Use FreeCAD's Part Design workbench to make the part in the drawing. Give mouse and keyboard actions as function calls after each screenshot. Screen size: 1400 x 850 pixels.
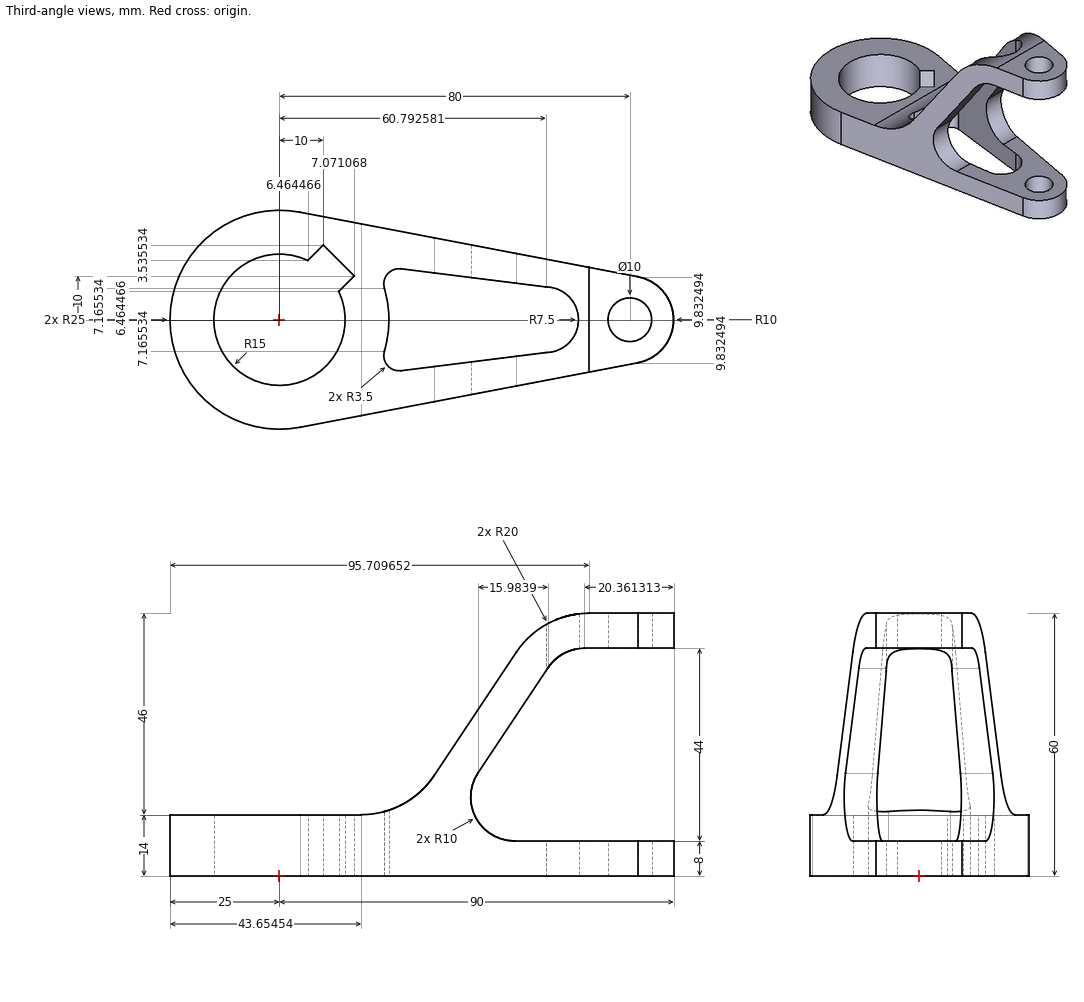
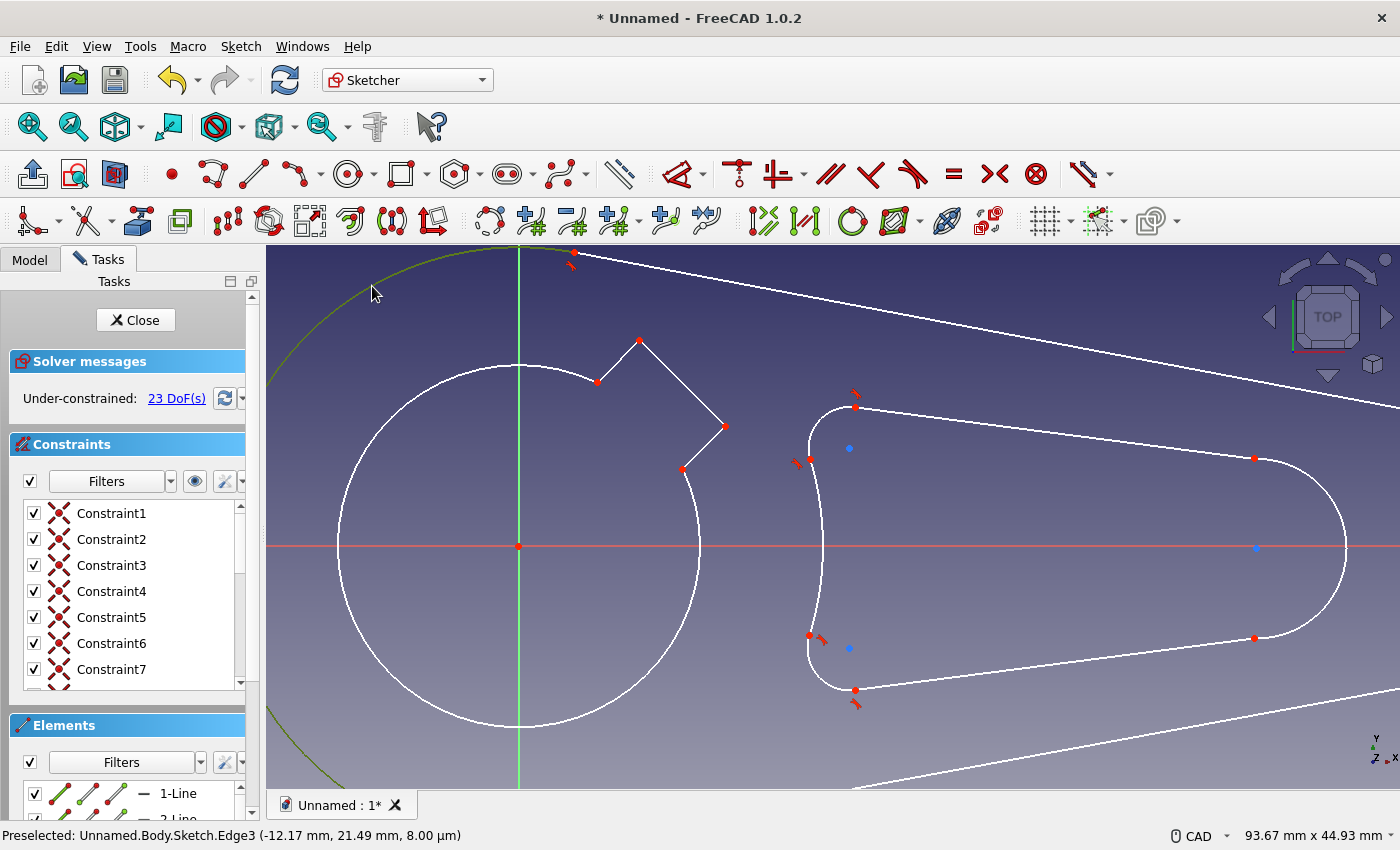
click(821, 583)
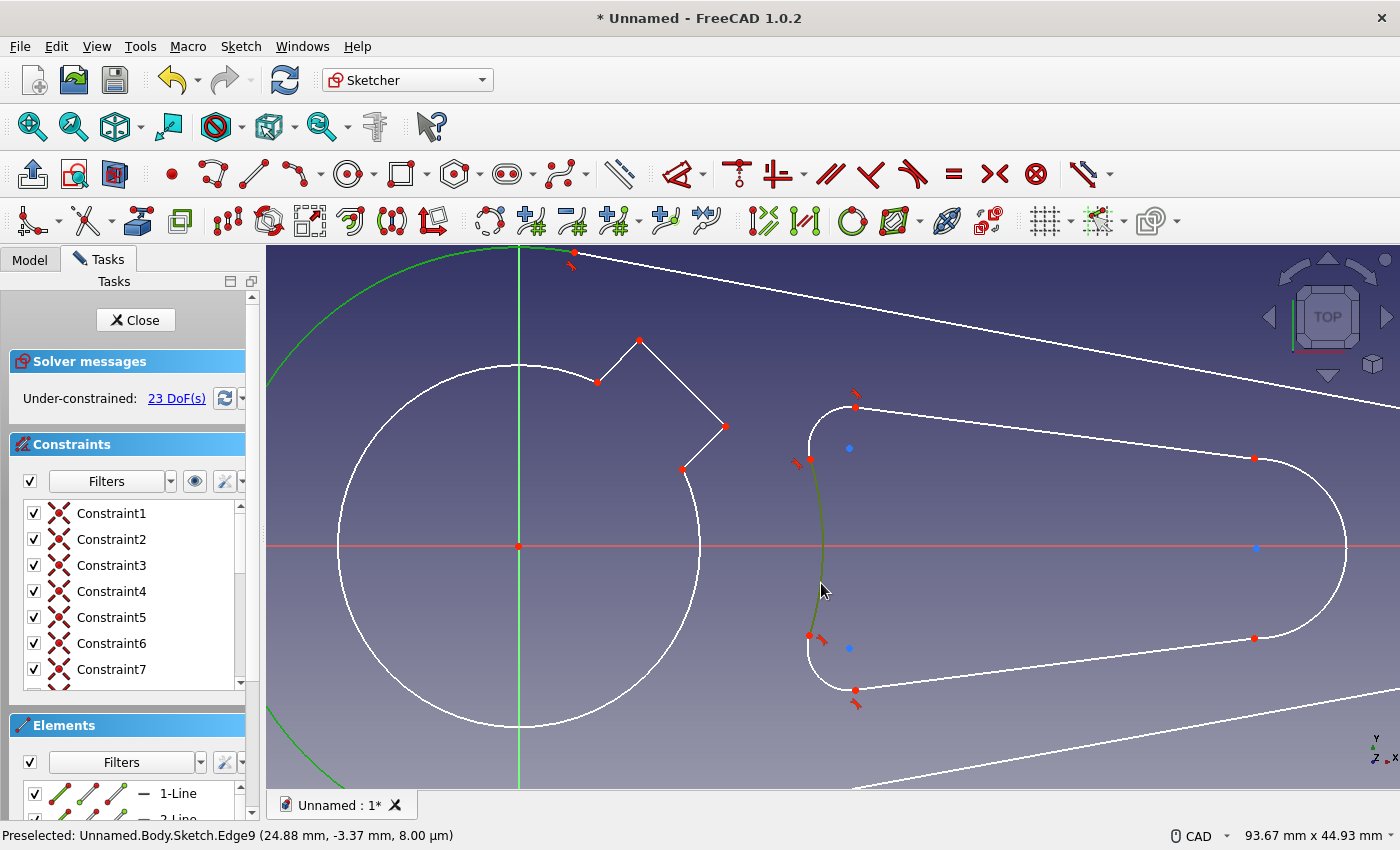
key(e)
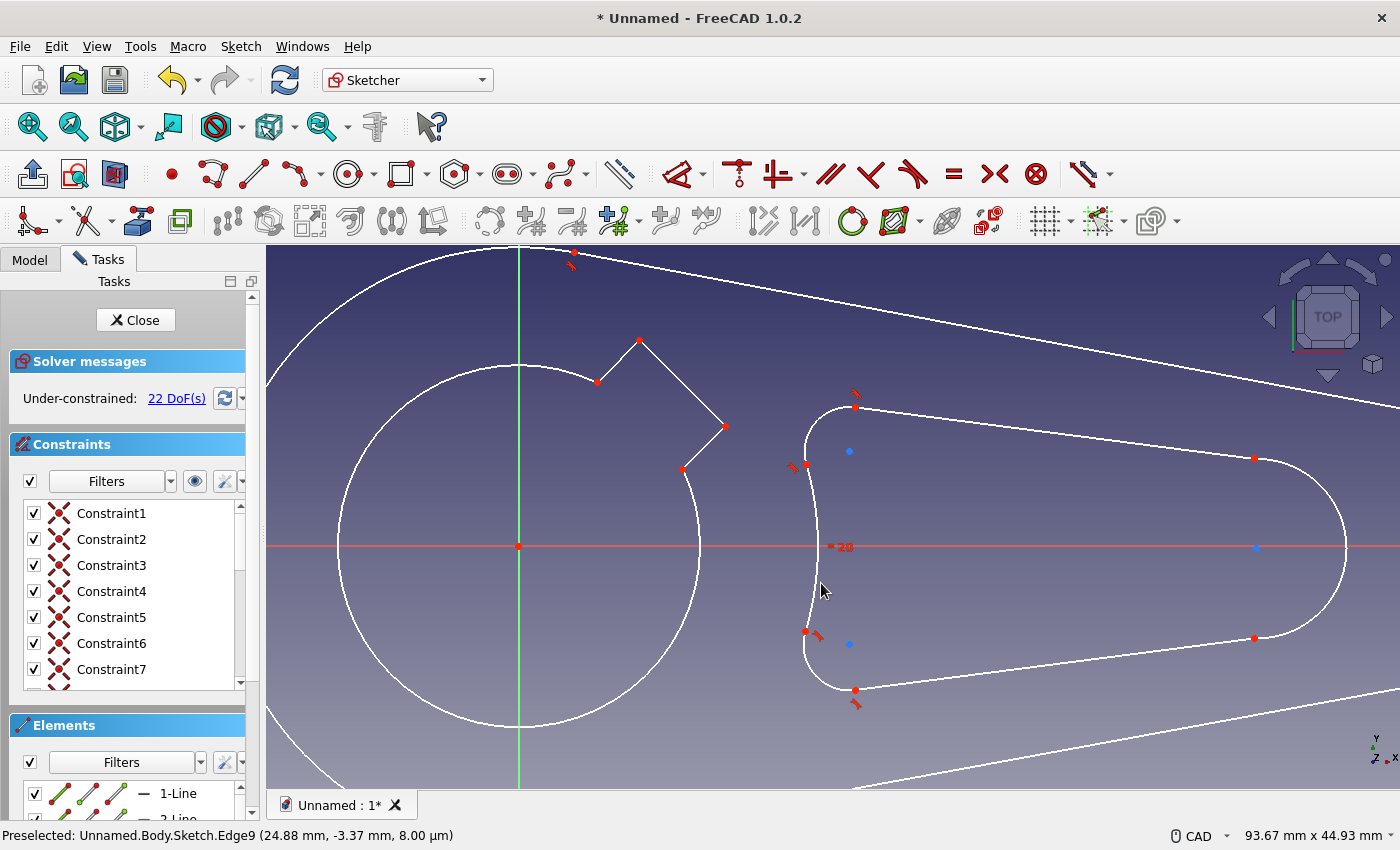
click(806, 658)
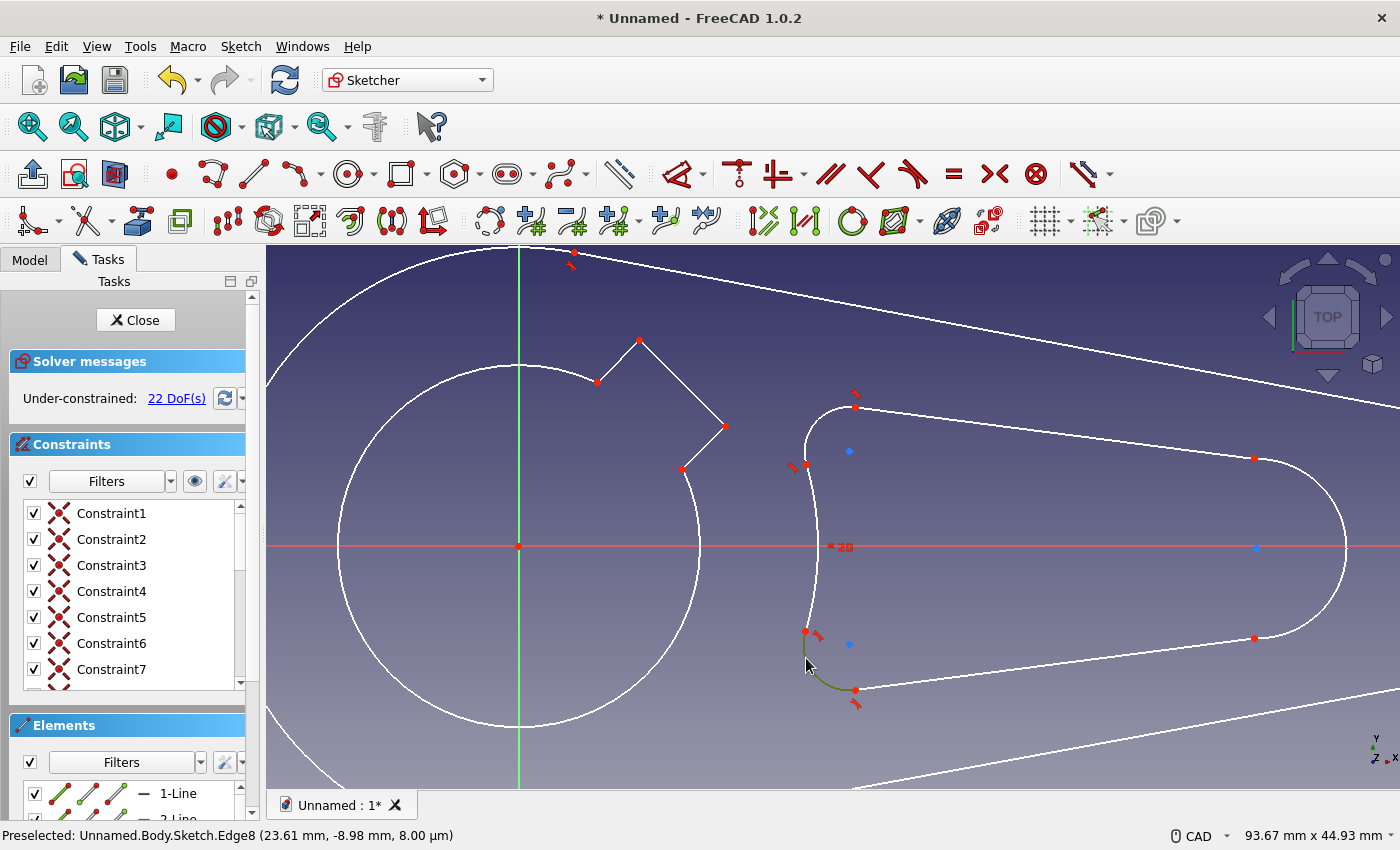
click(829, 412)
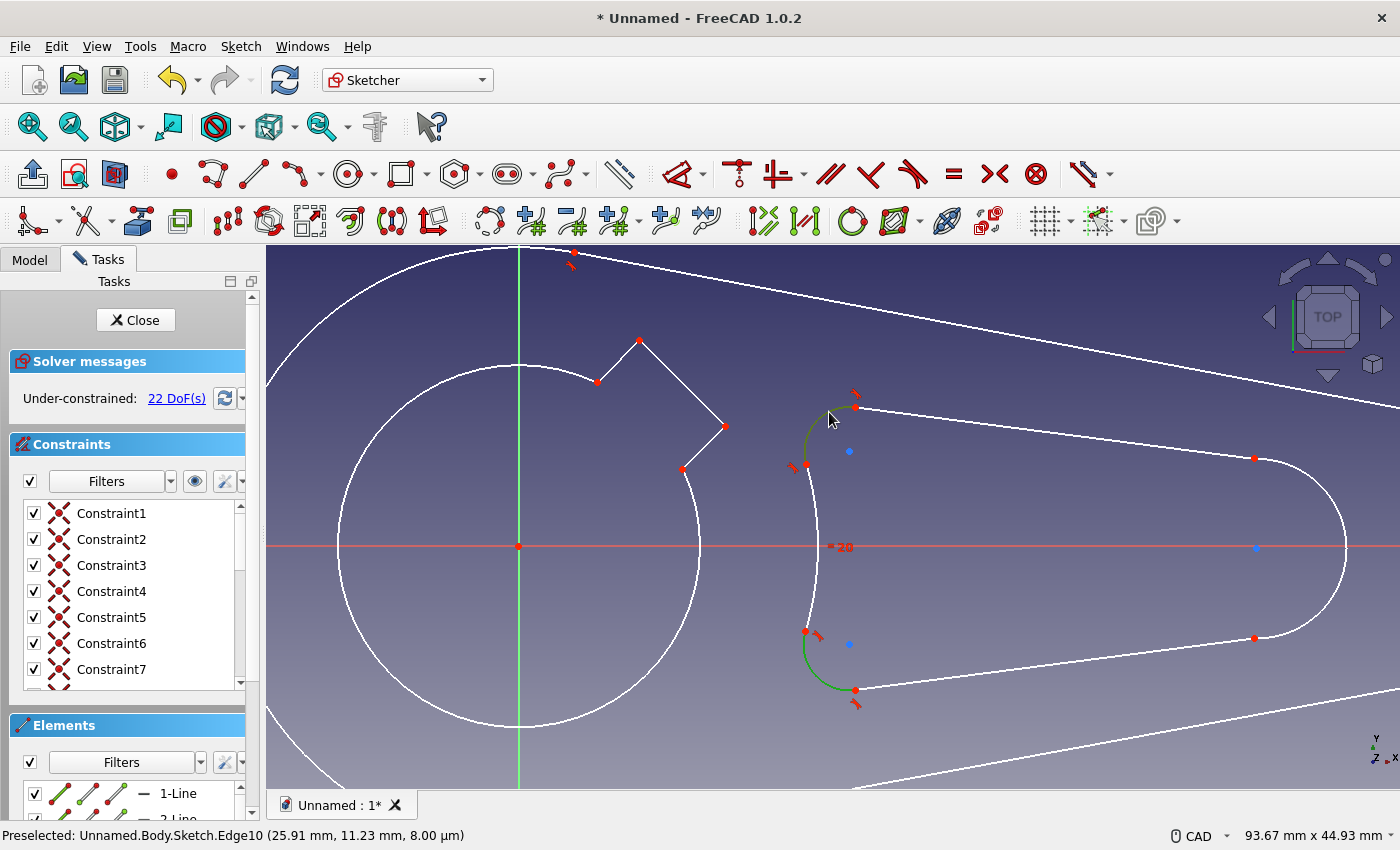
click(954, 174)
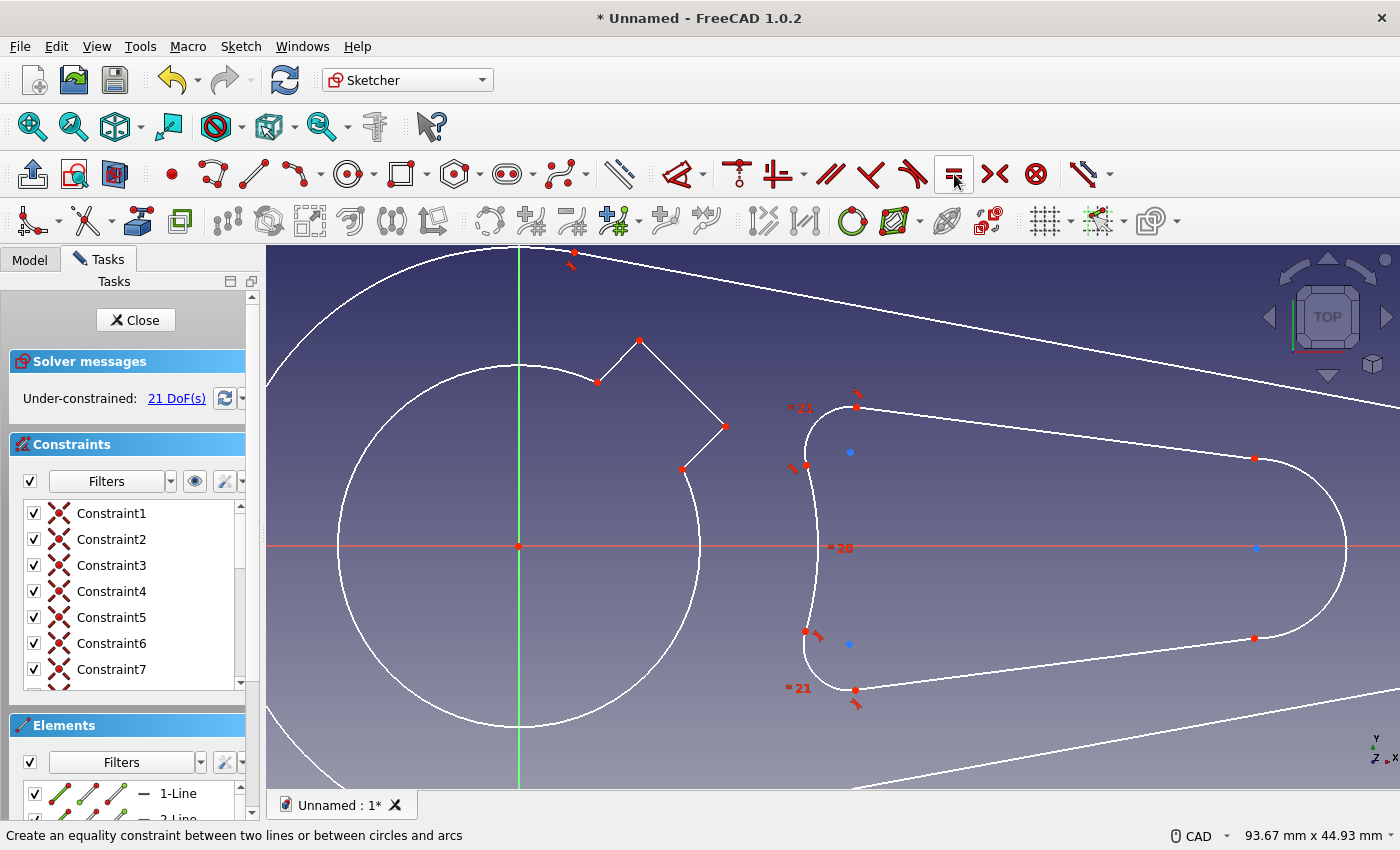
scroll(644, 493, down, 4)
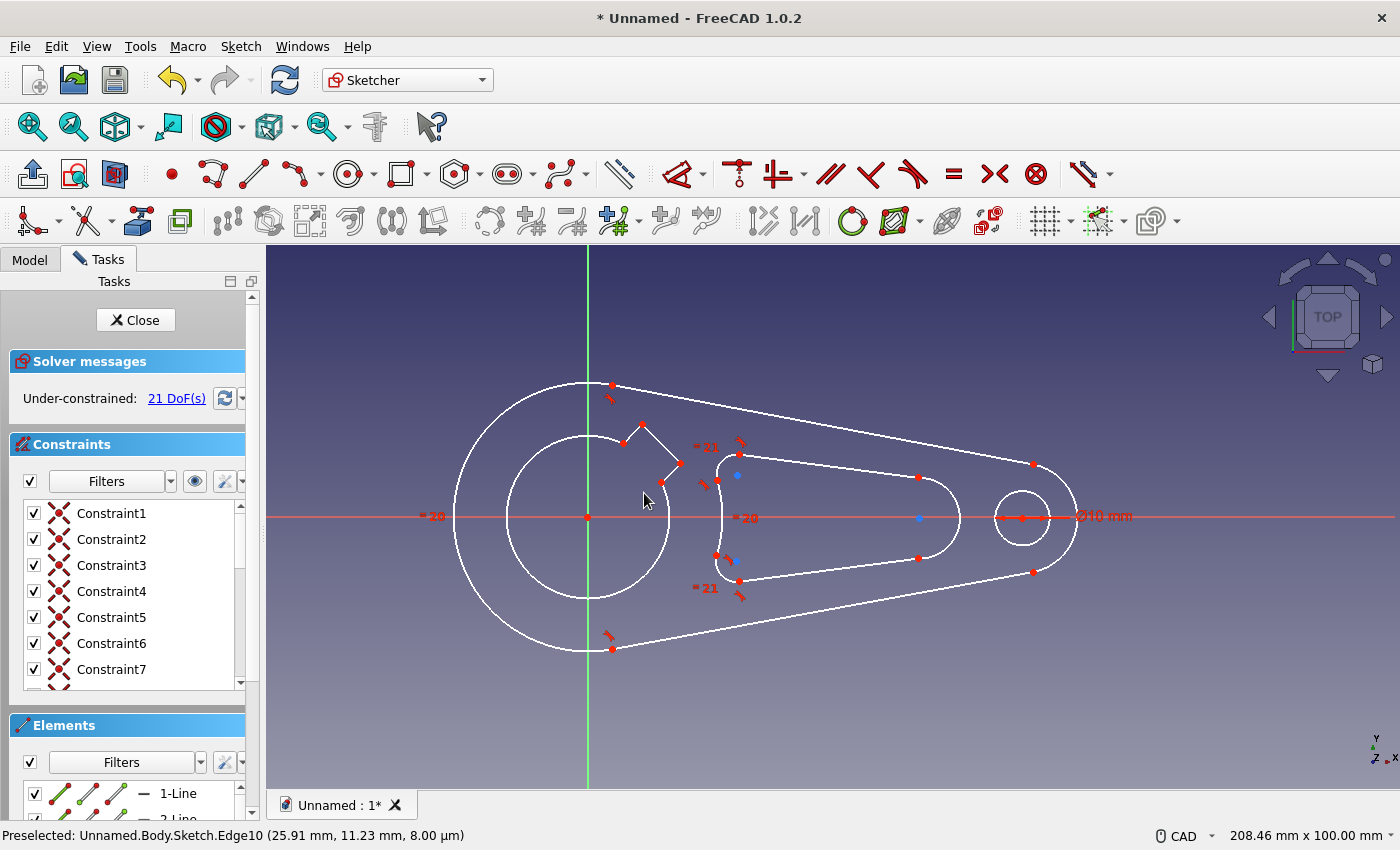
click(1023, 518)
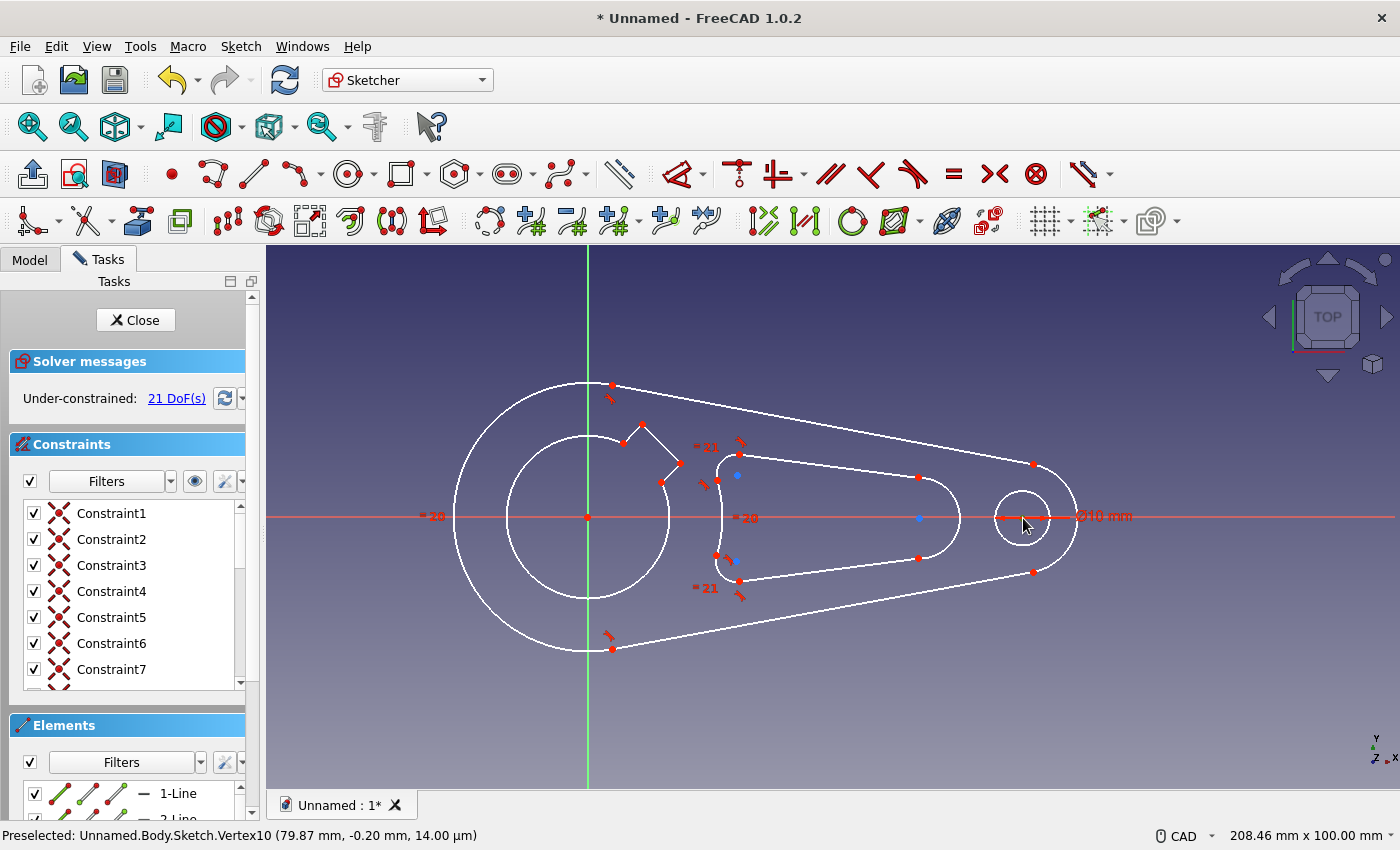
click(361, 517)